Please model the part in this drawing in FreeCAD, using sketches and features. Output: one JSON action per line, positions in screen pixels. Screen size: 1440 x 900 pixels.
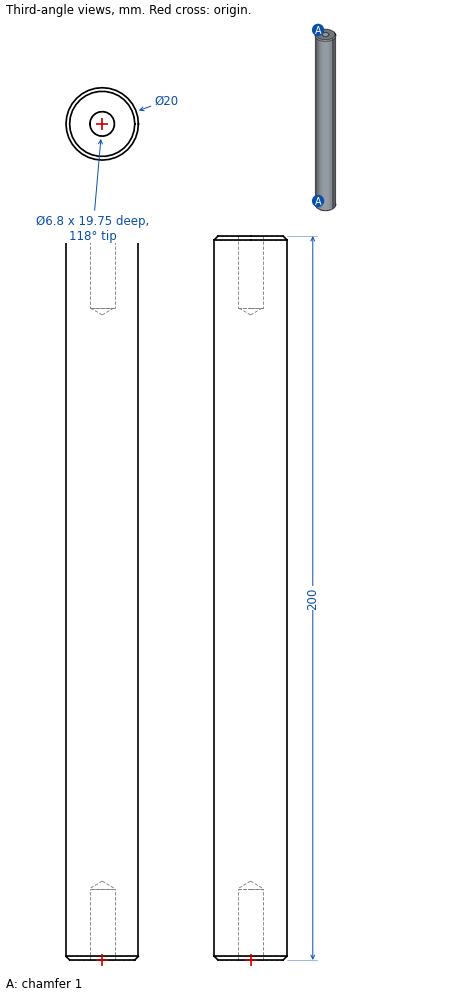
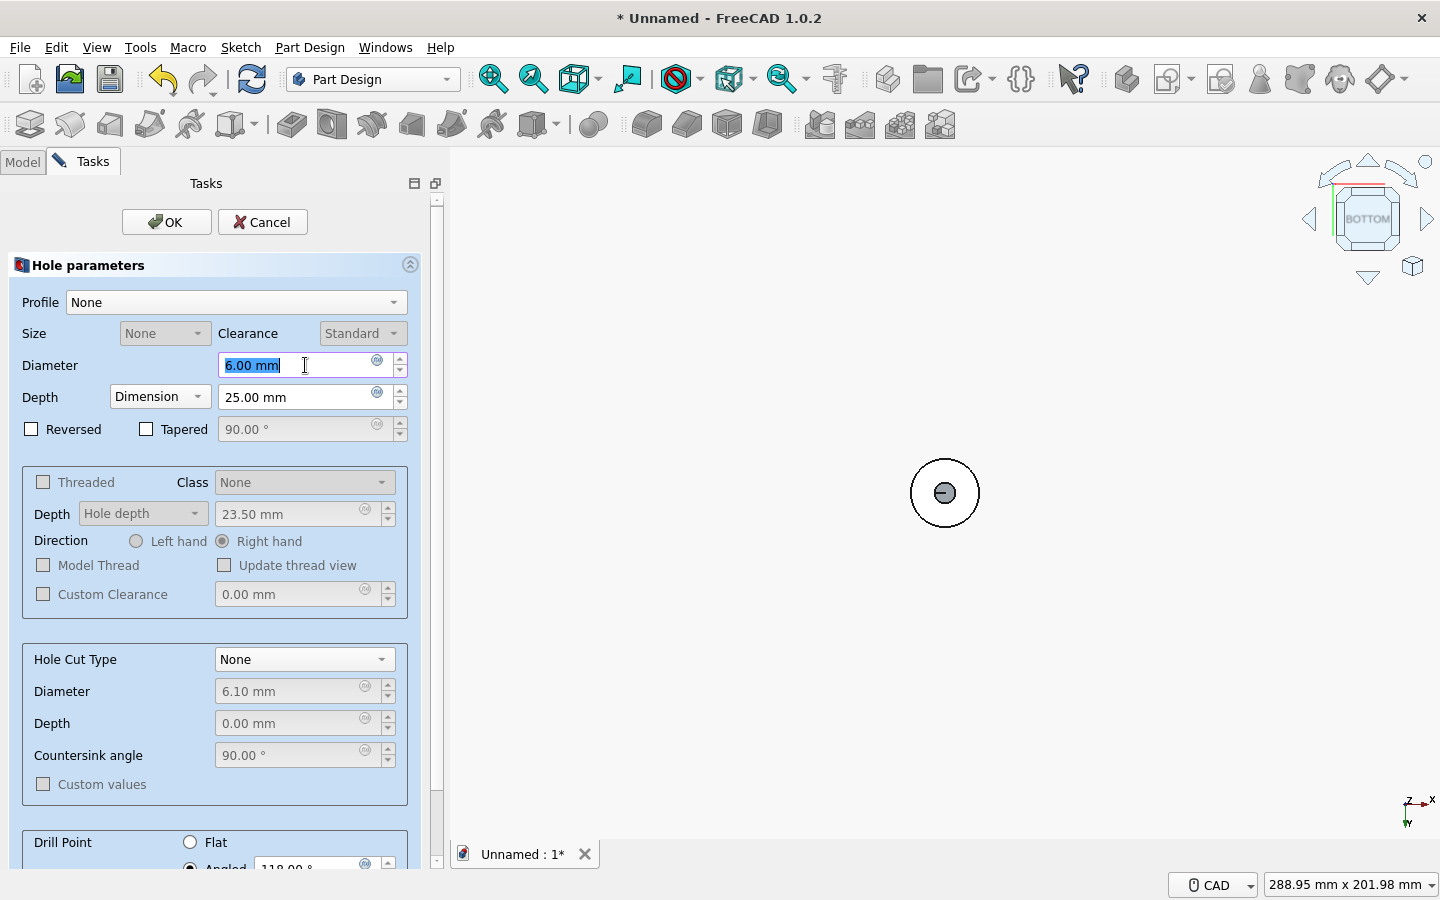
{"action": "type", "text": "6.8"}
{"action": "key", "text": "Tab"}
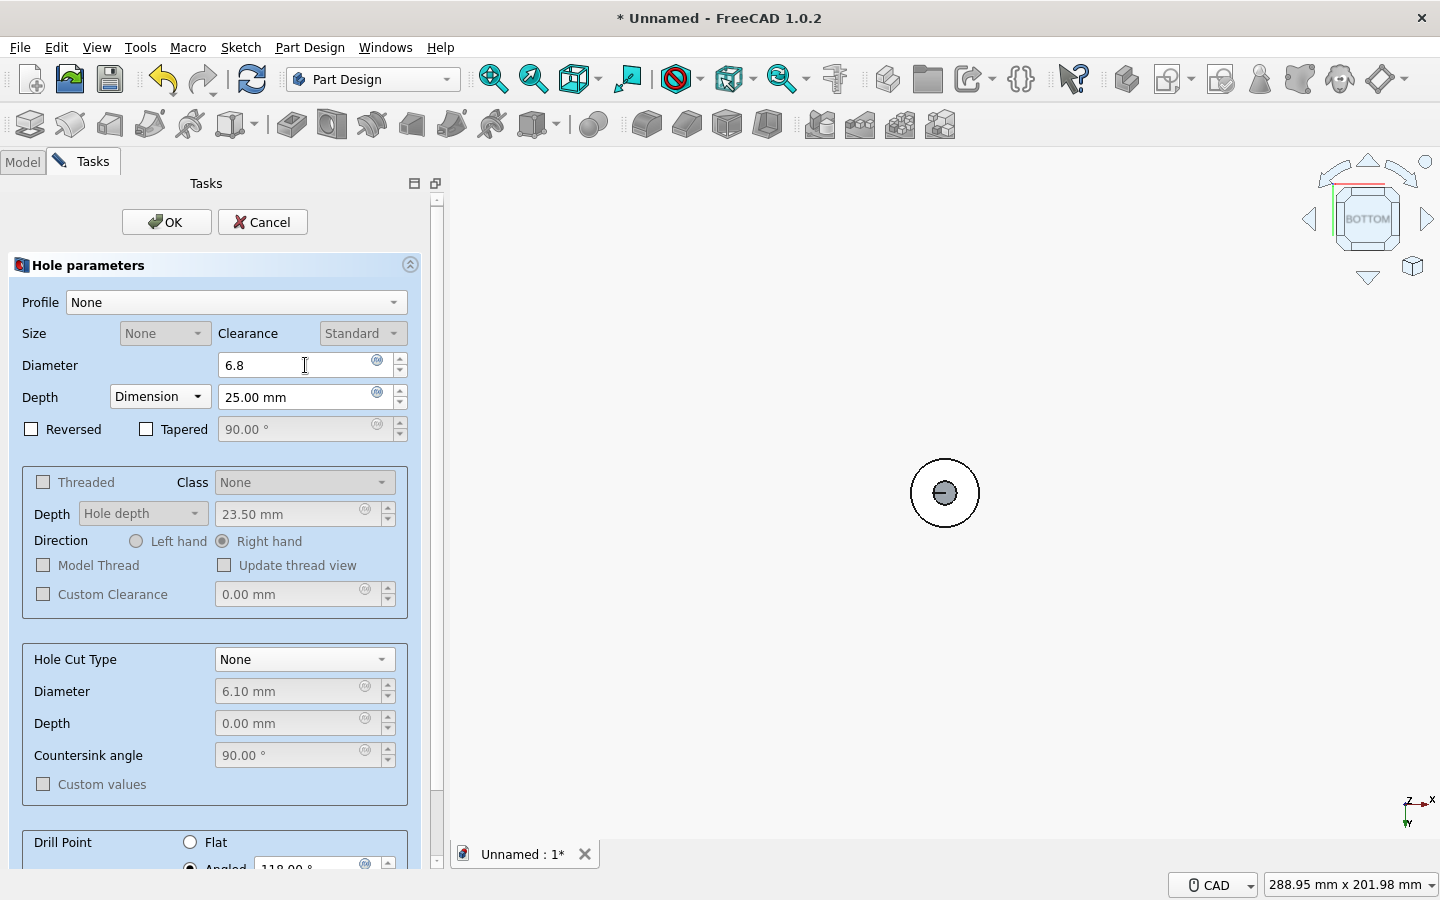
{"action": "triple_click", "coordinate": [305, 397]}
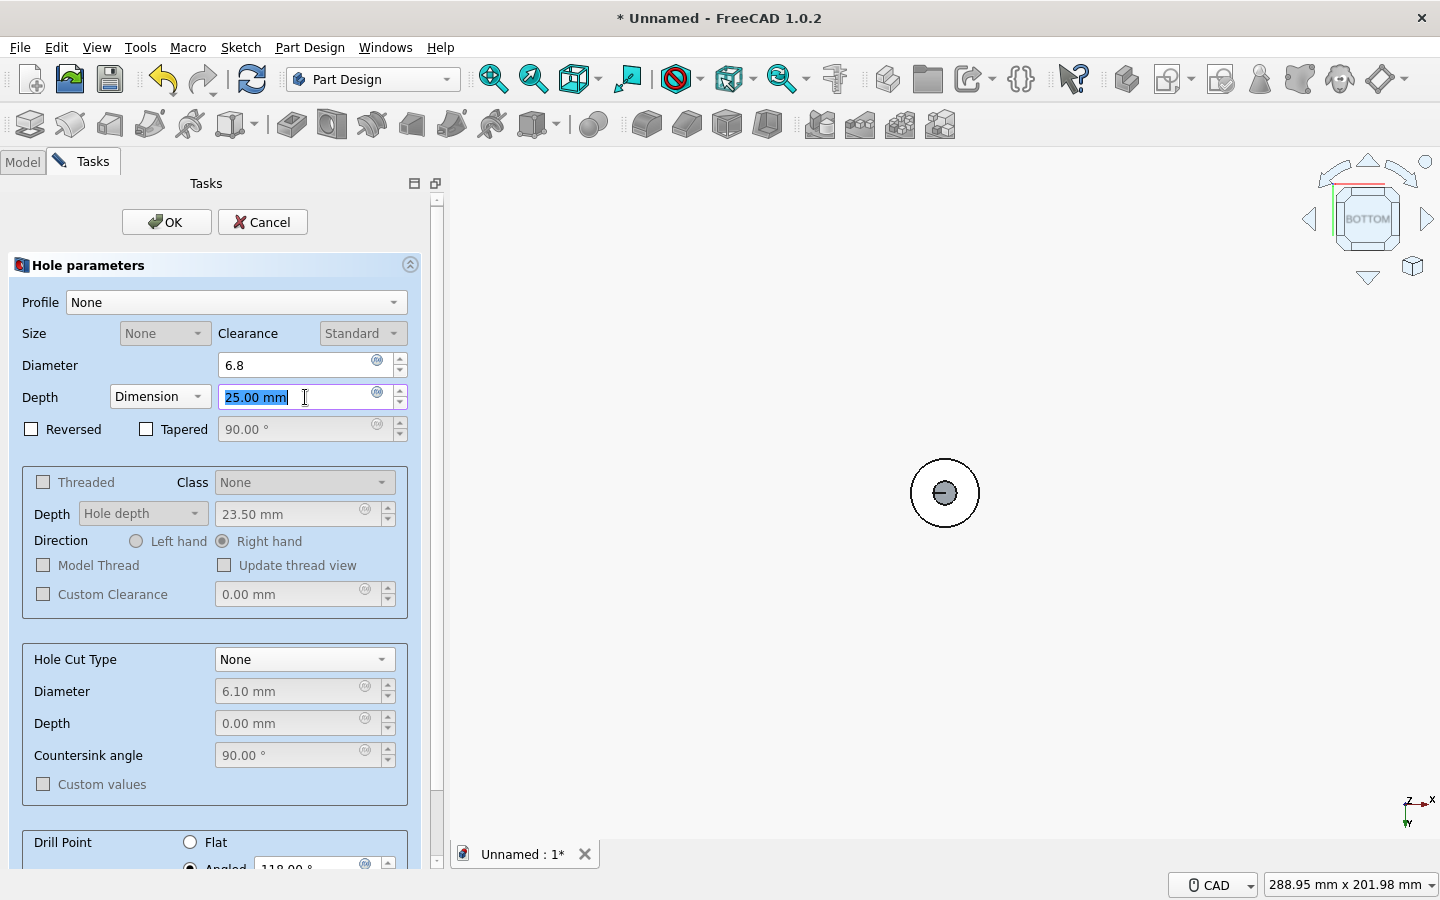
{"action": "type", "text": "19.75"}
{"action": "key", "text": "Tab"}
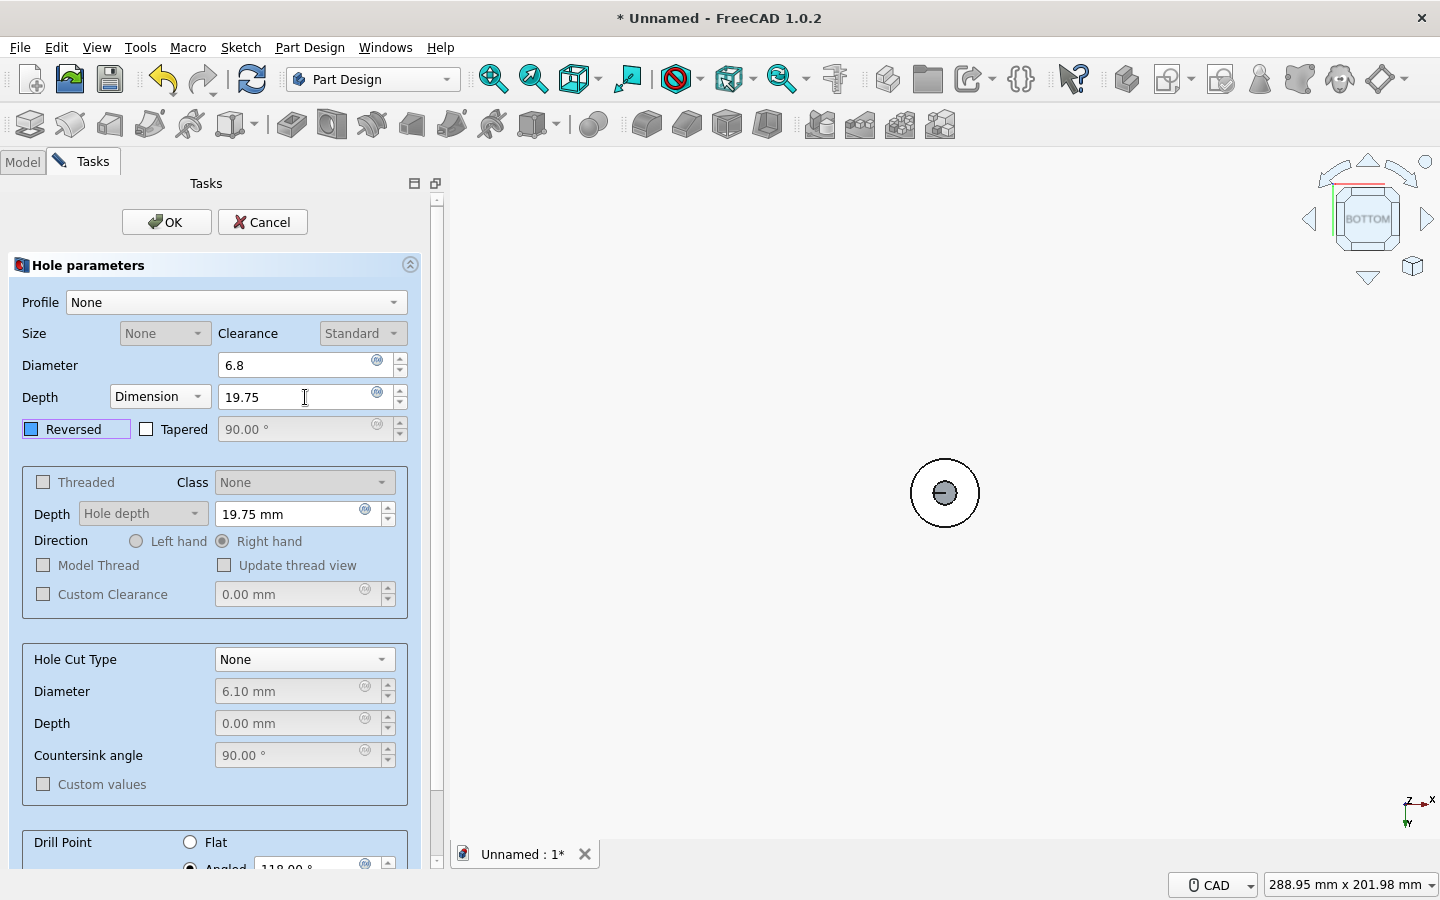
{"action": "left_click", "coordinate": [167, 222]}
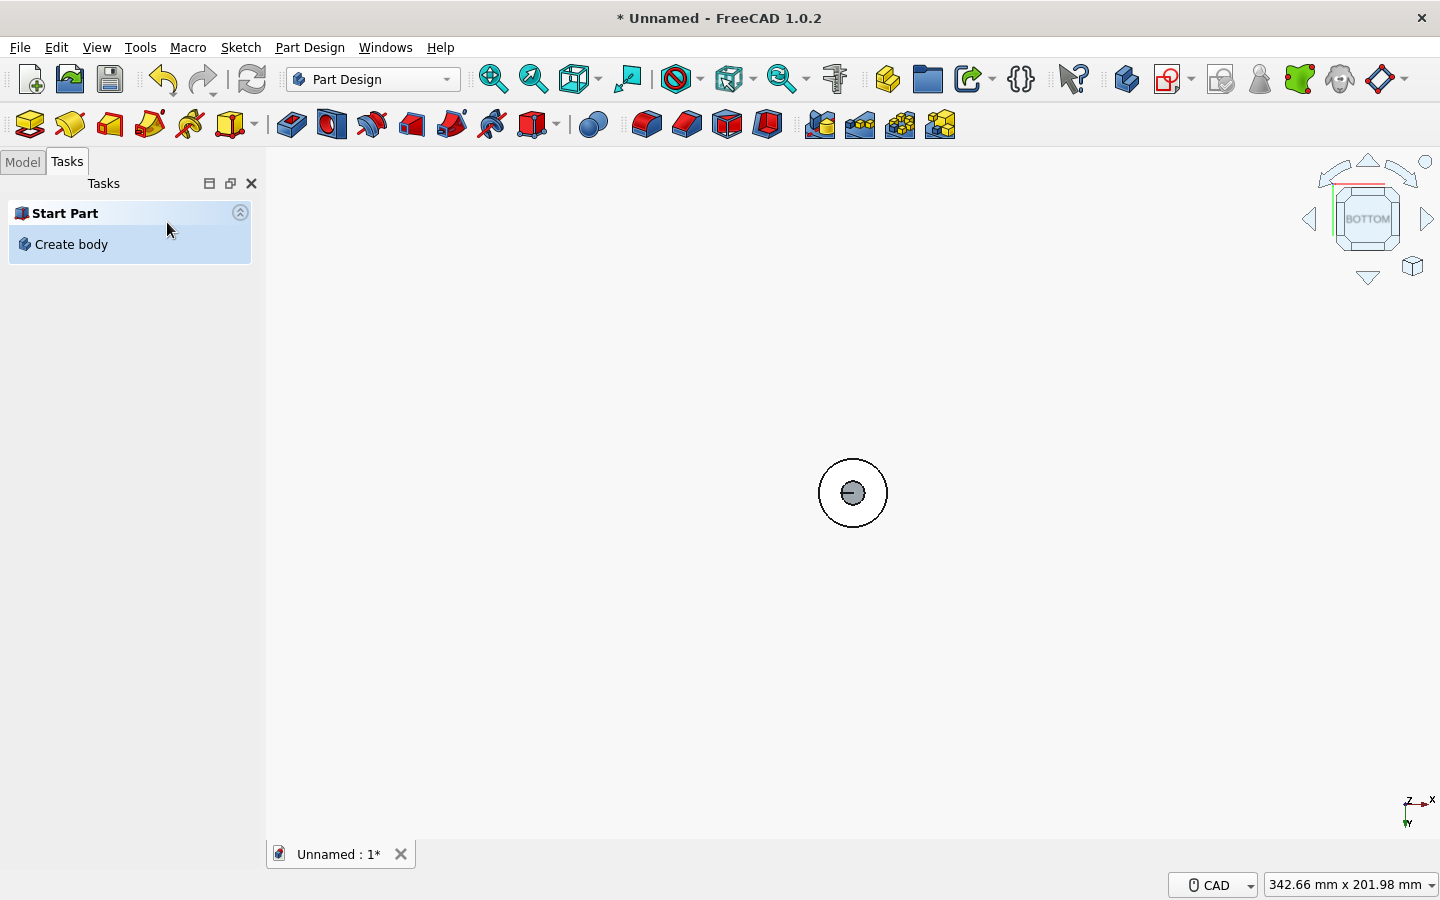
{"action": "key", "text": "v f"}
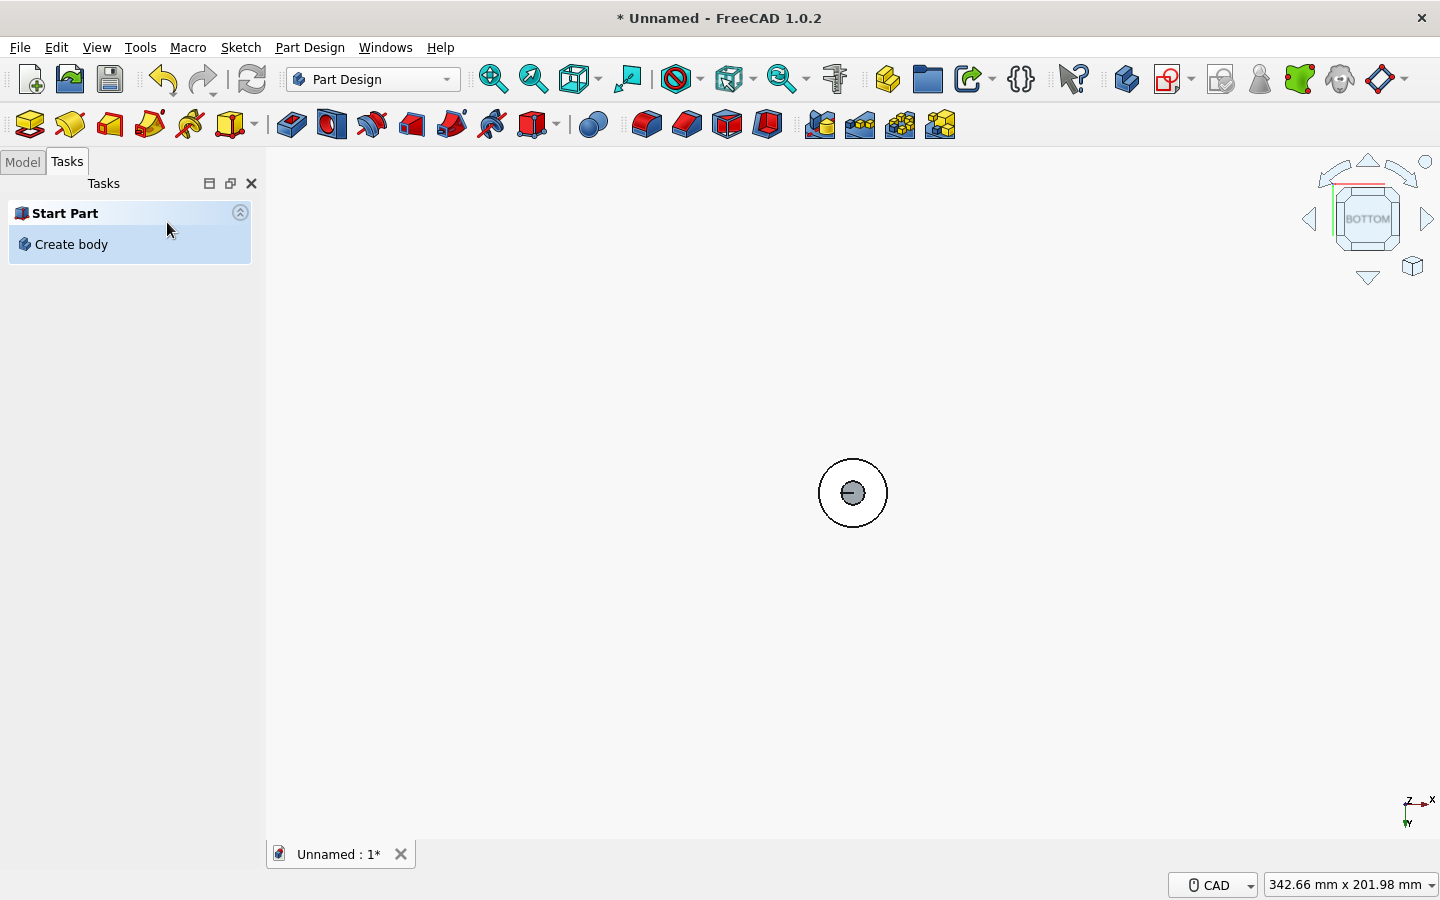
{"action": "key", "text": "0"}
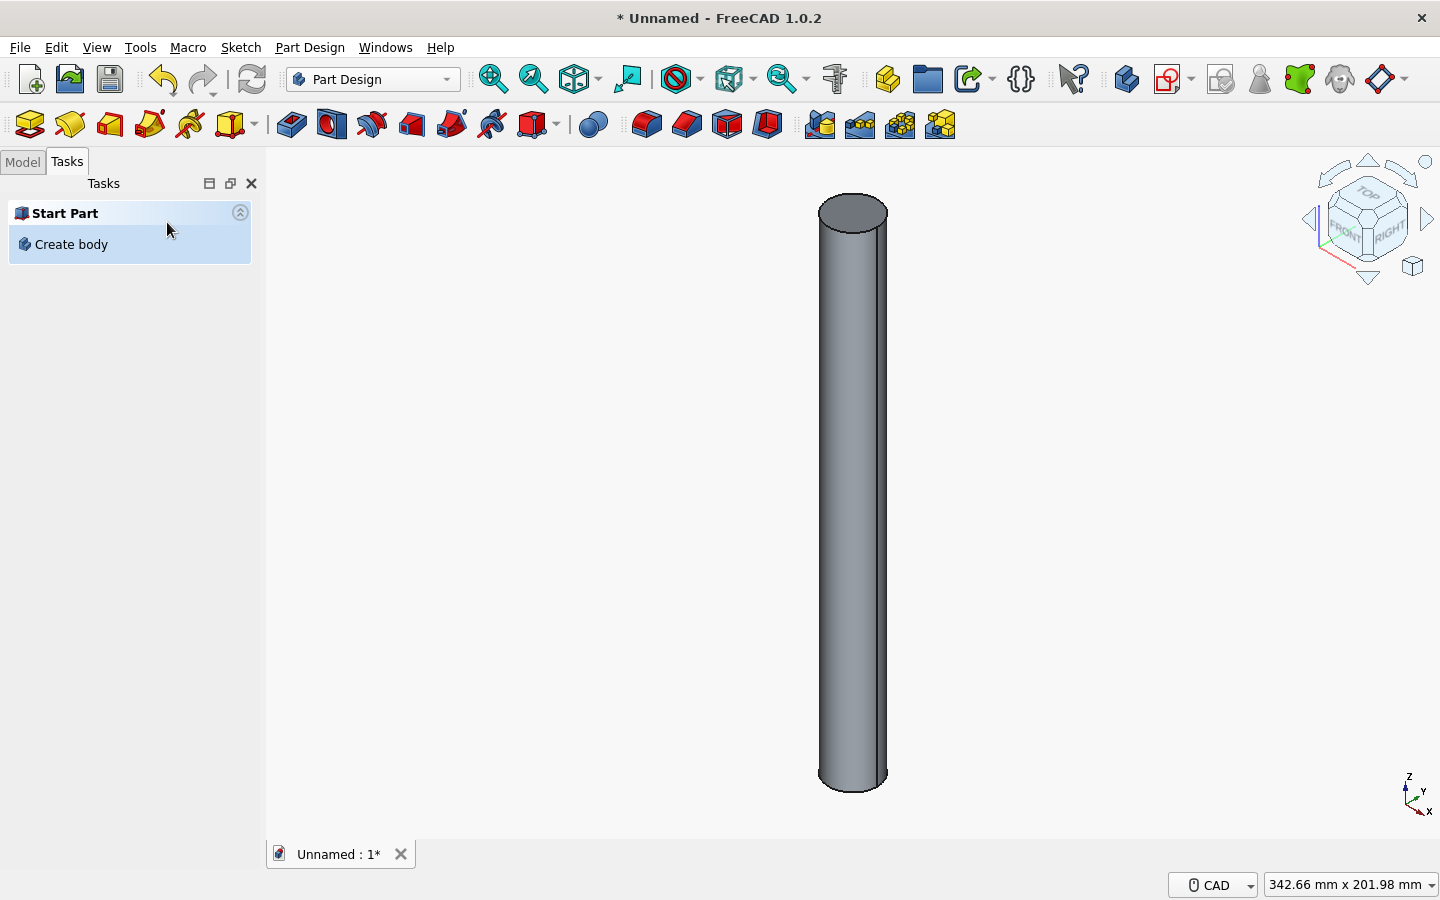
{"action": "left_click", "coordinate": [853, 212]}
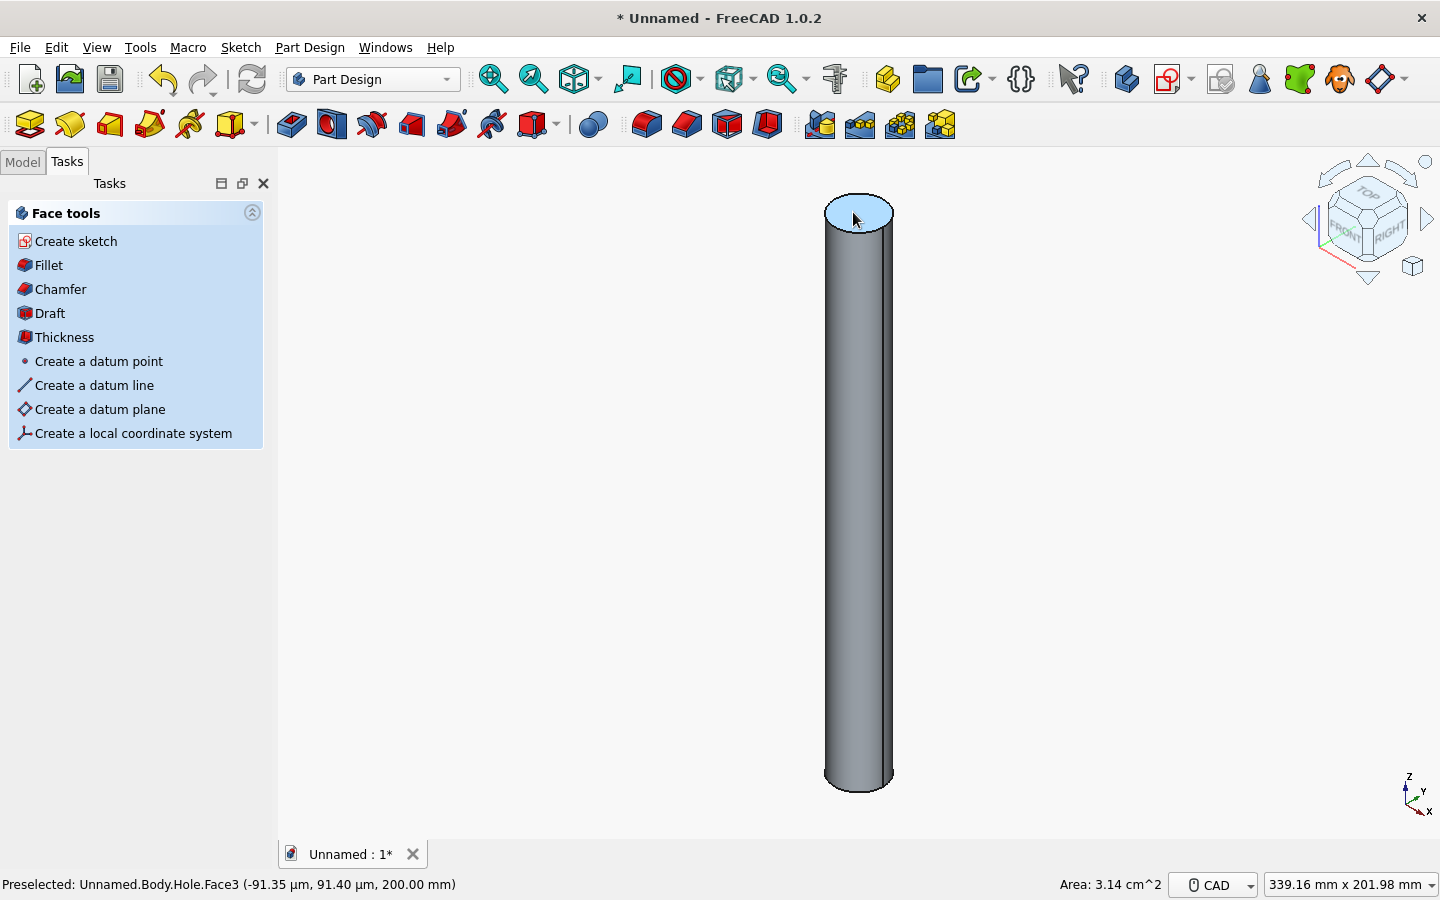
{"action": "left_click", "coordinate": [1168, 80]}